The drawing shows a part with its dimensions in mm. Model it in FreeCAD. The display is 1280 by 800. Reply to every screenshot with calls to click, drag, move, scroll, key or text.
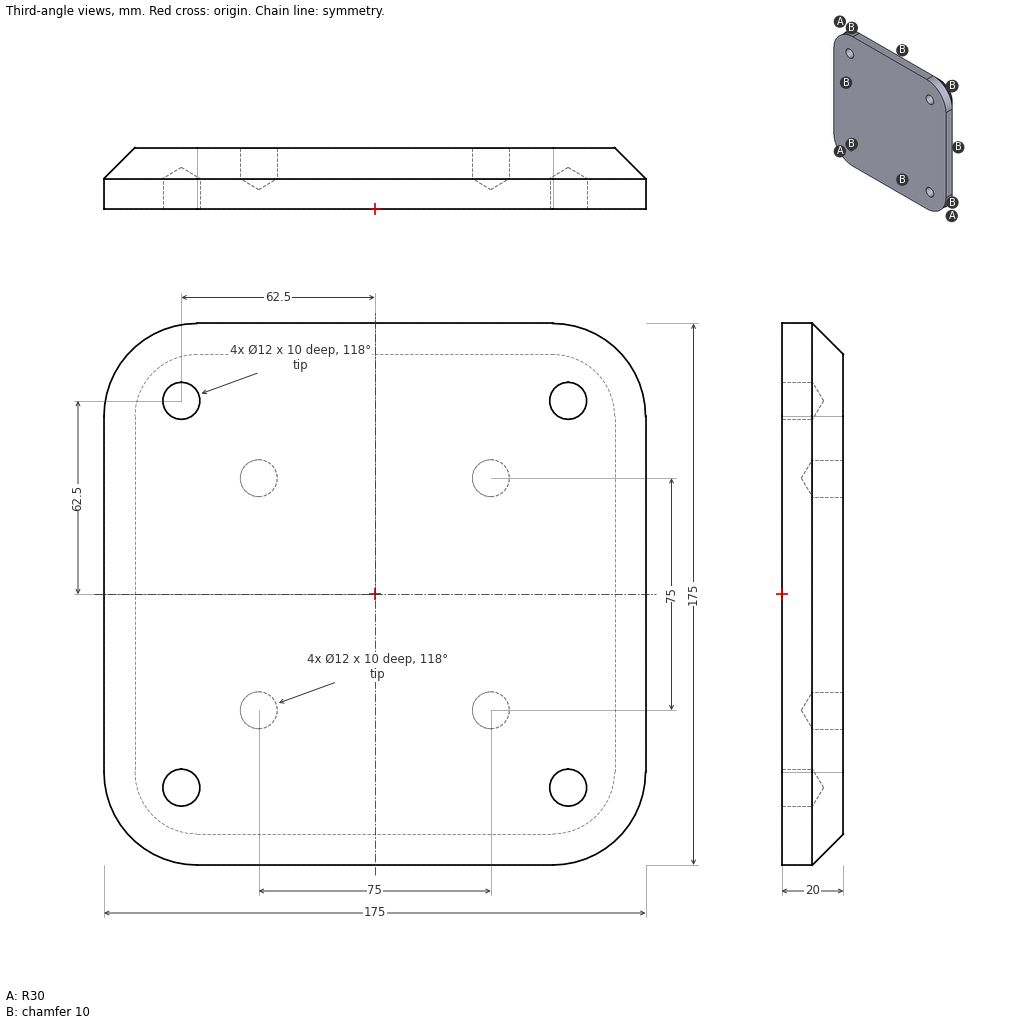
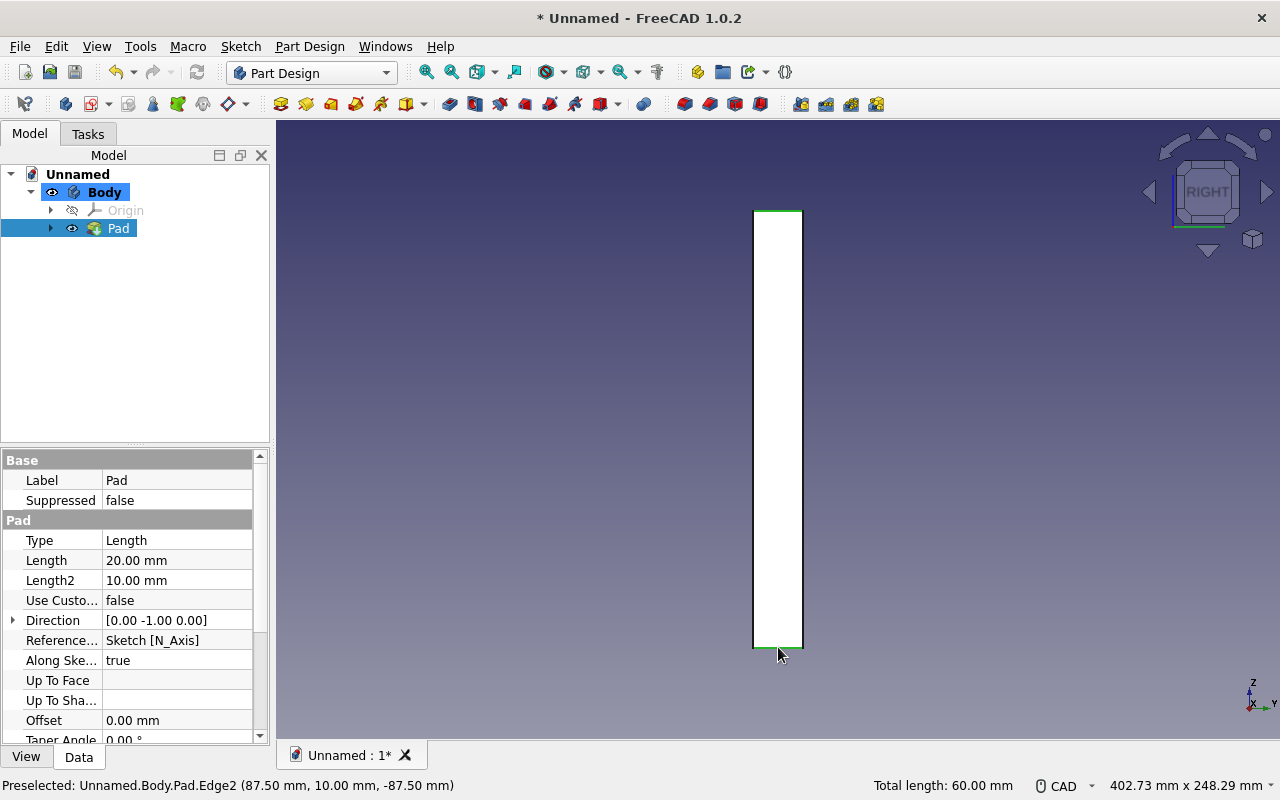
key(5)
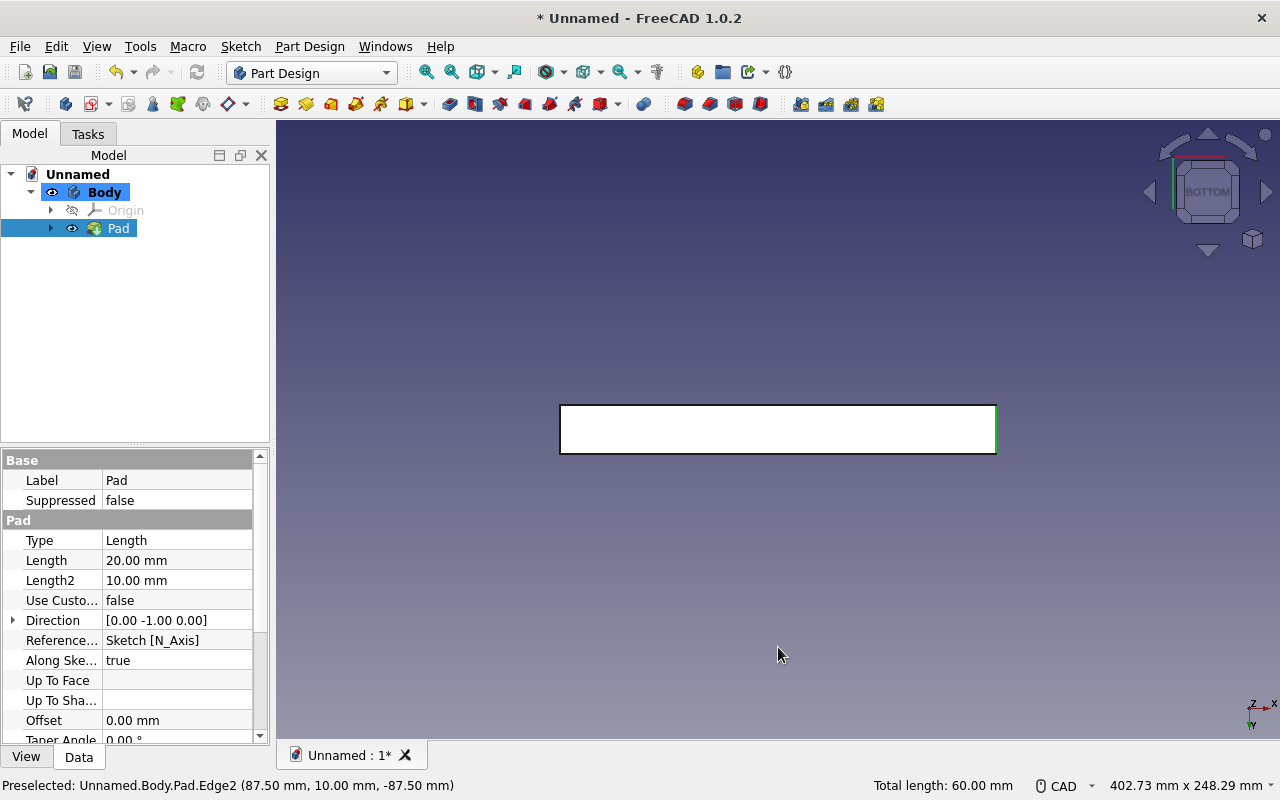
click(427, 72)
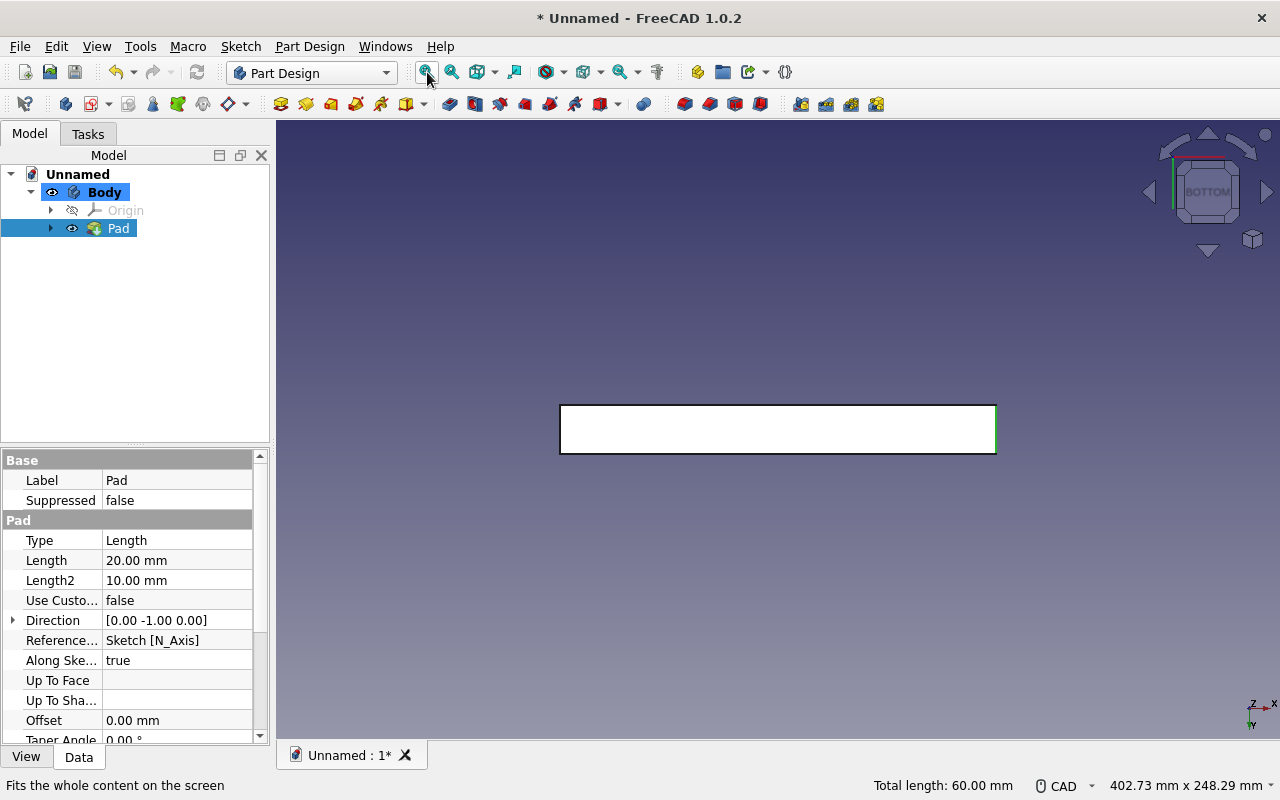
click(560, 428, ctrl)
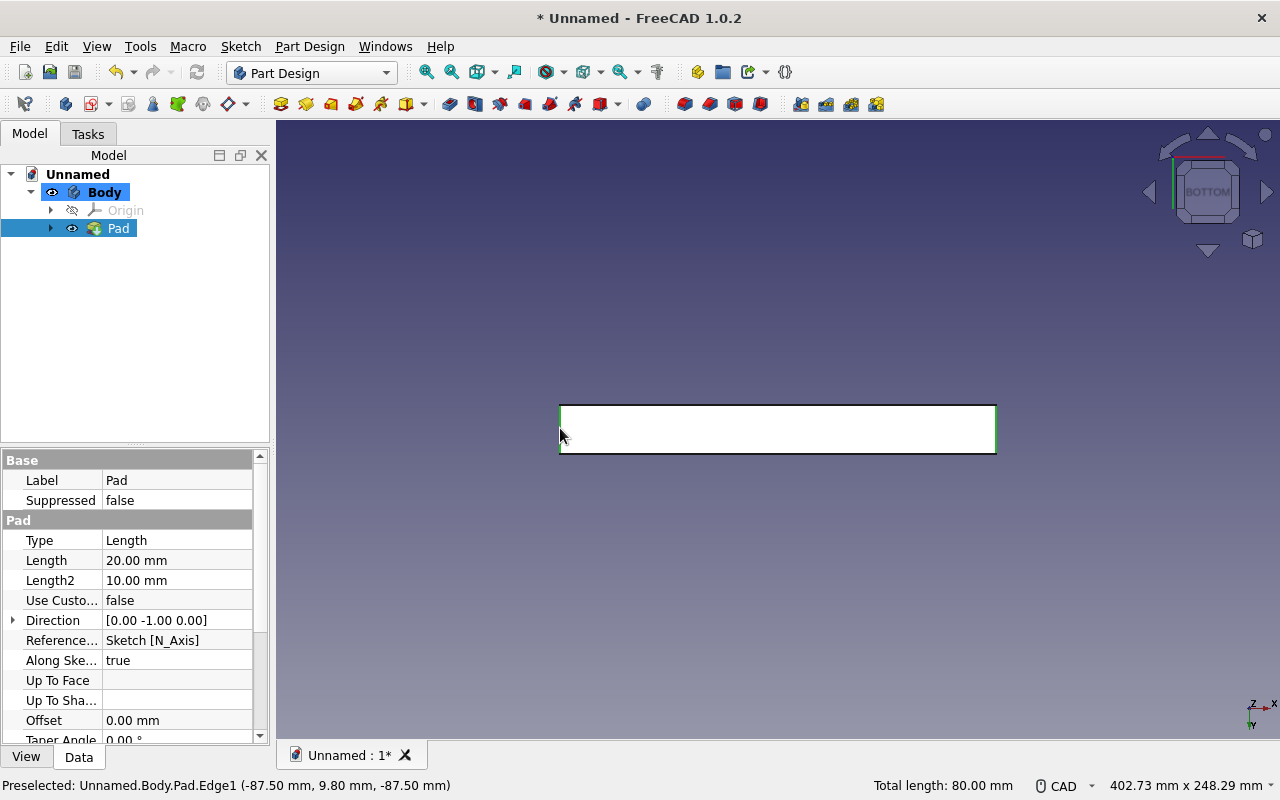
click(685, 104)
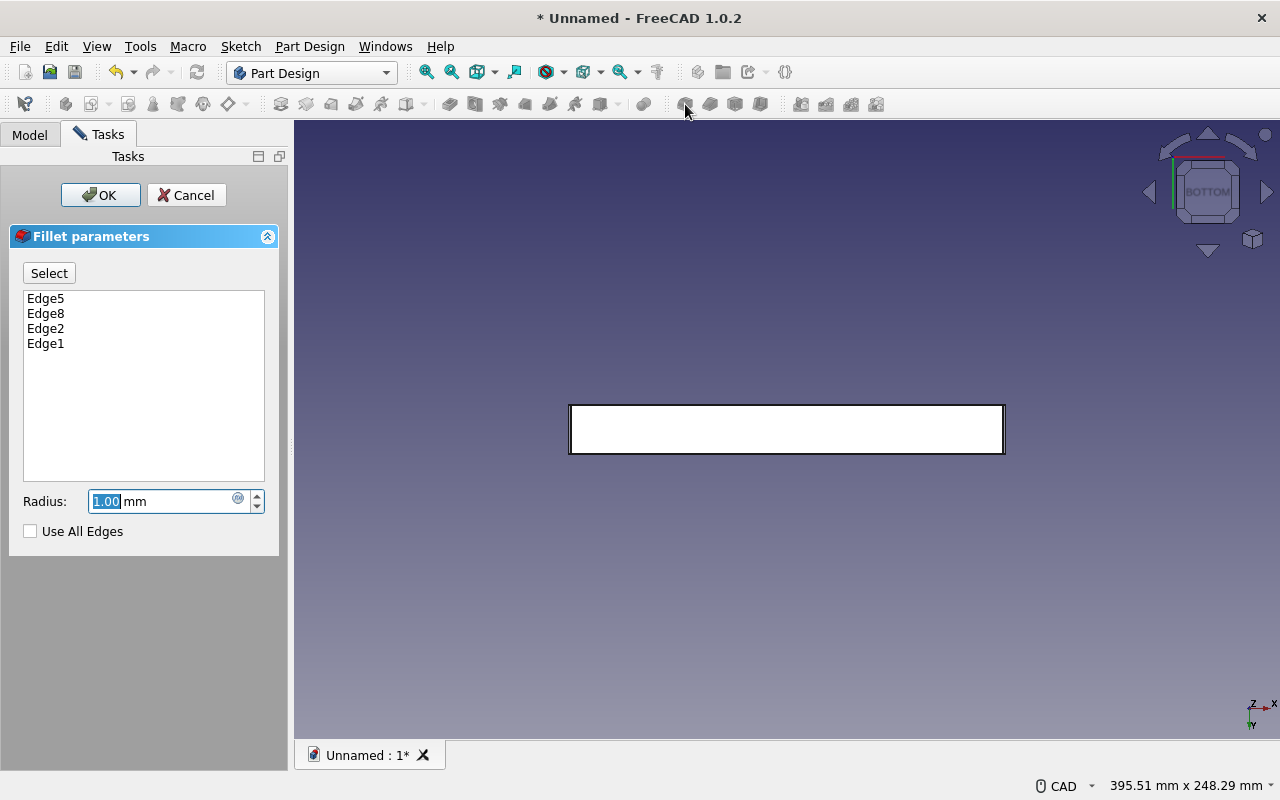
text(30)
key(Tab)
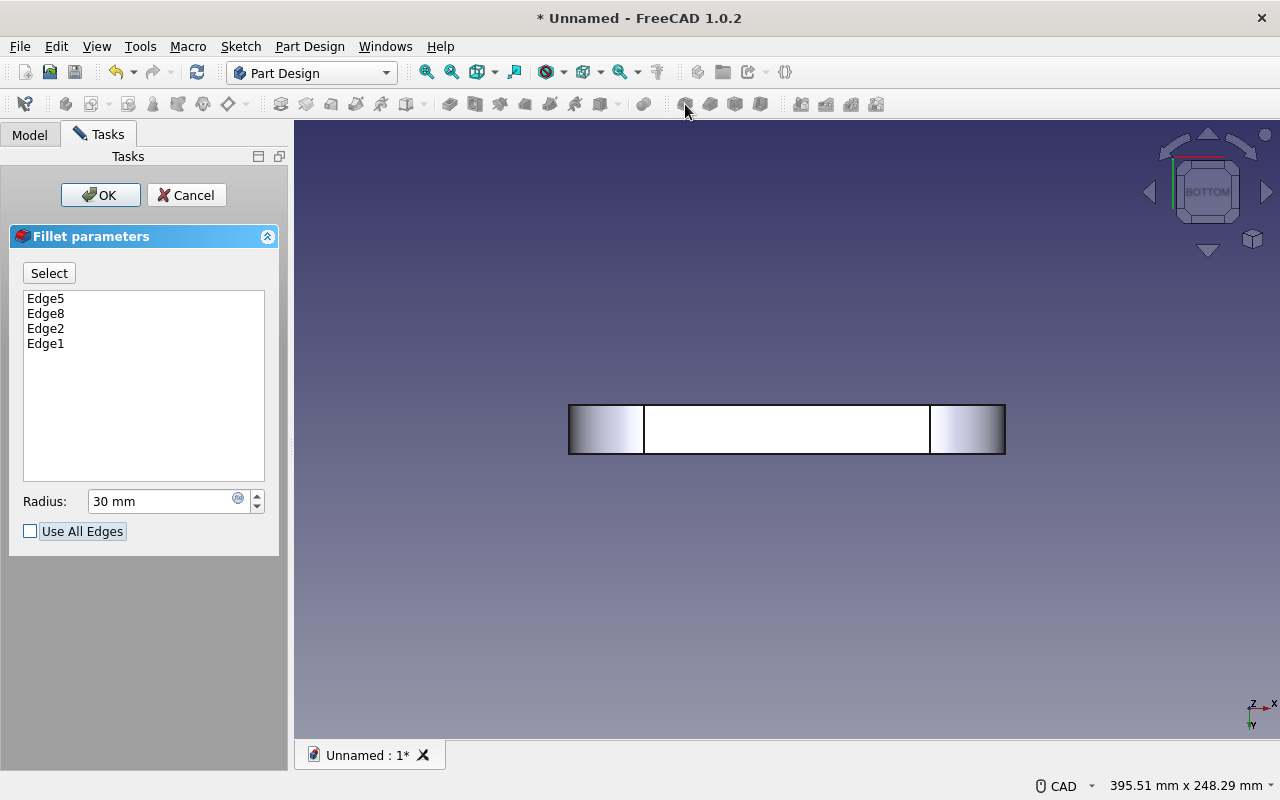
click(101, 195)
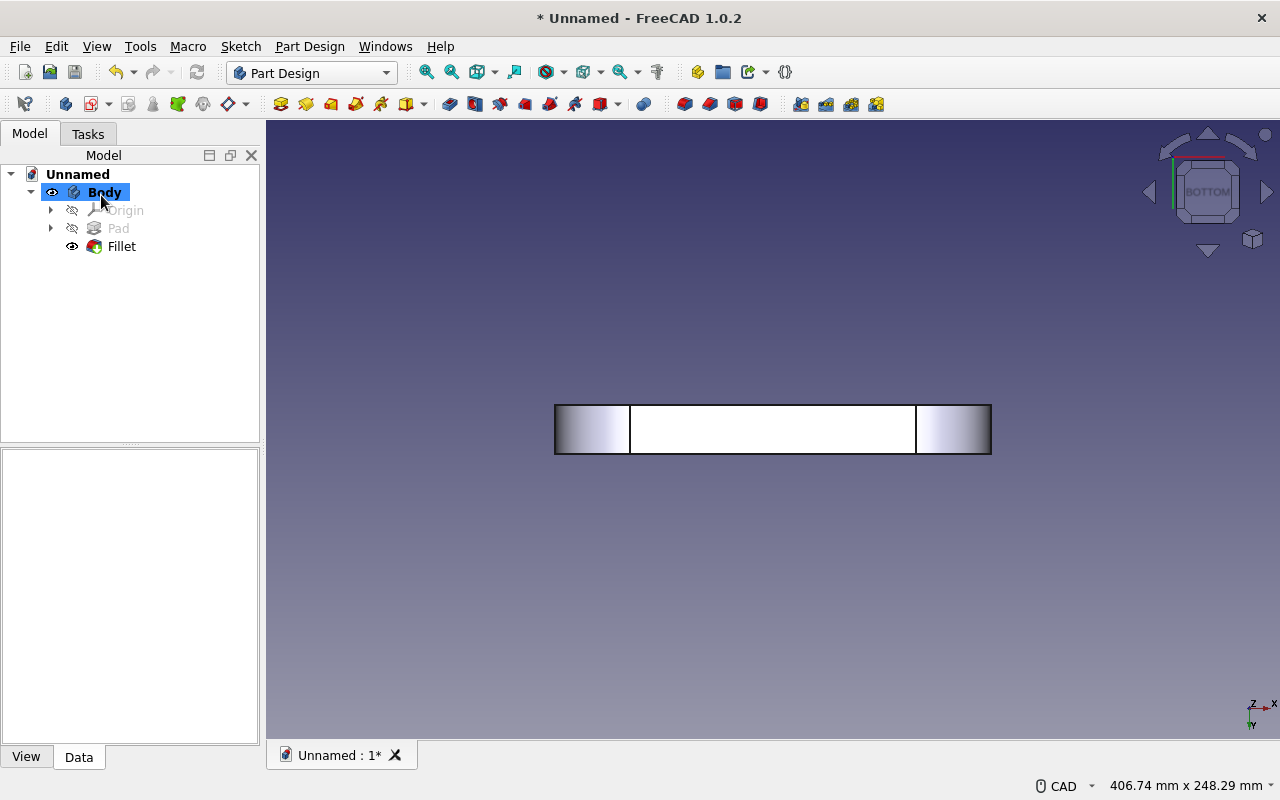
click(427, 72)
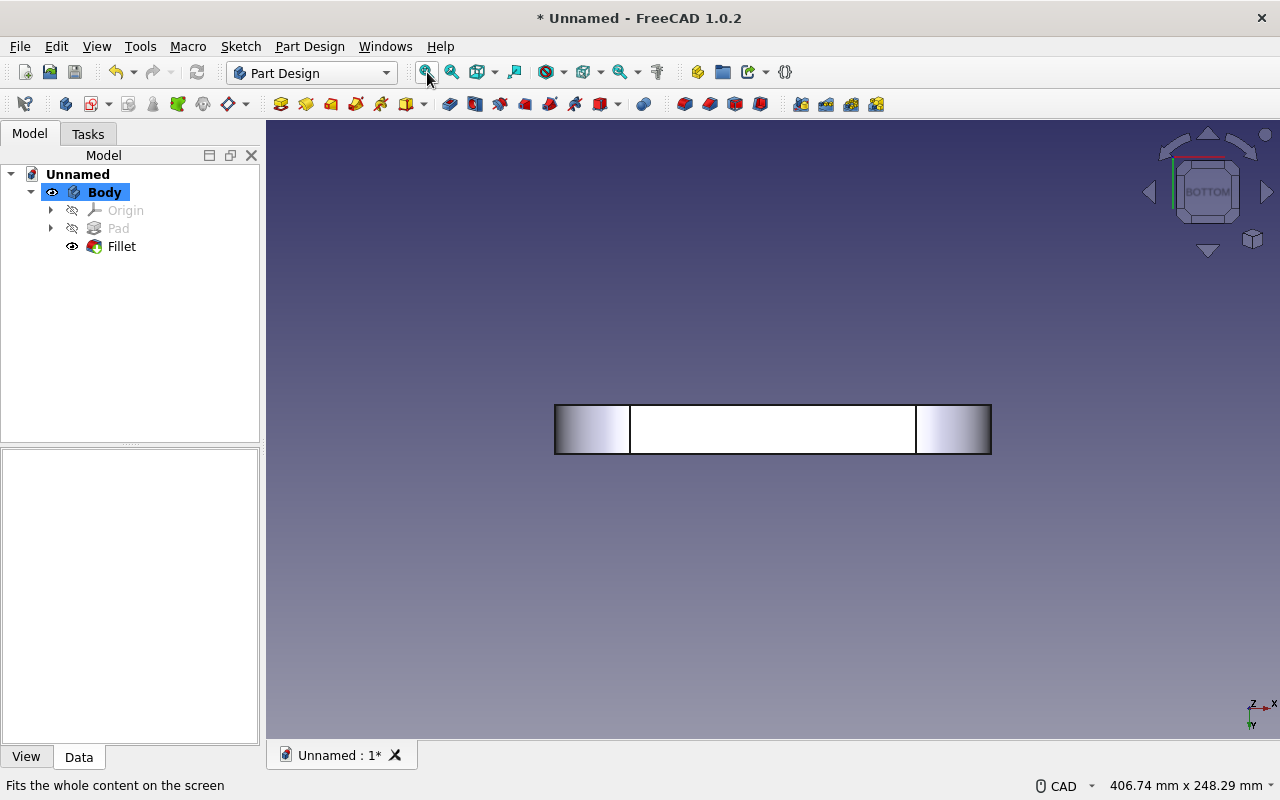
key(0)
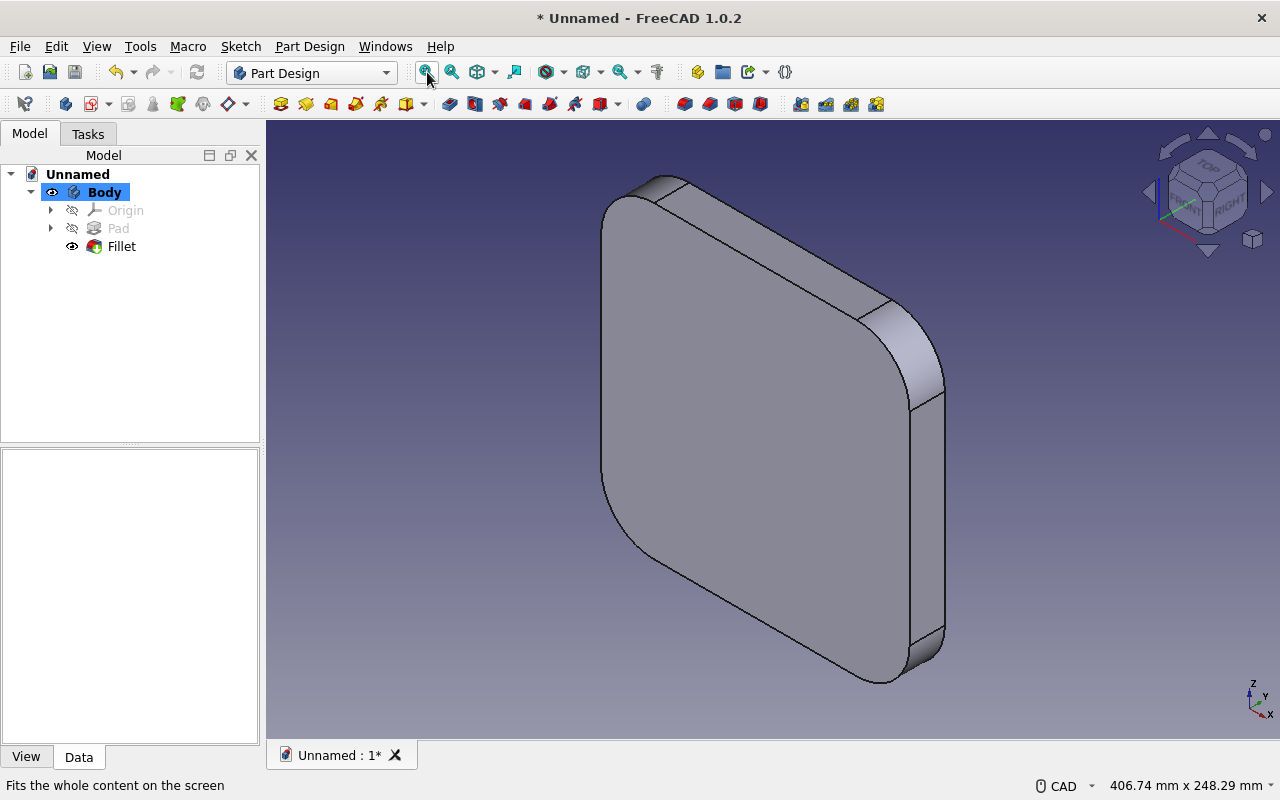
key(2)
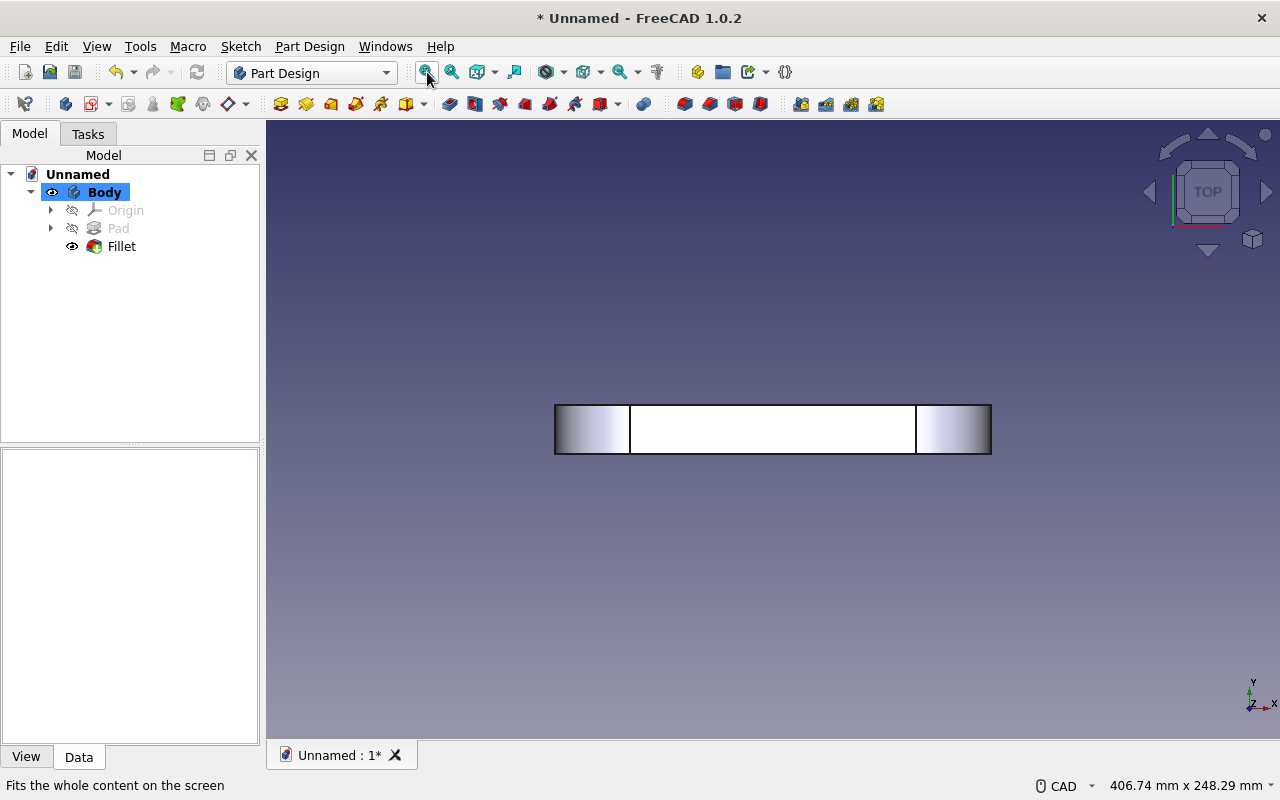
click(427, 72)